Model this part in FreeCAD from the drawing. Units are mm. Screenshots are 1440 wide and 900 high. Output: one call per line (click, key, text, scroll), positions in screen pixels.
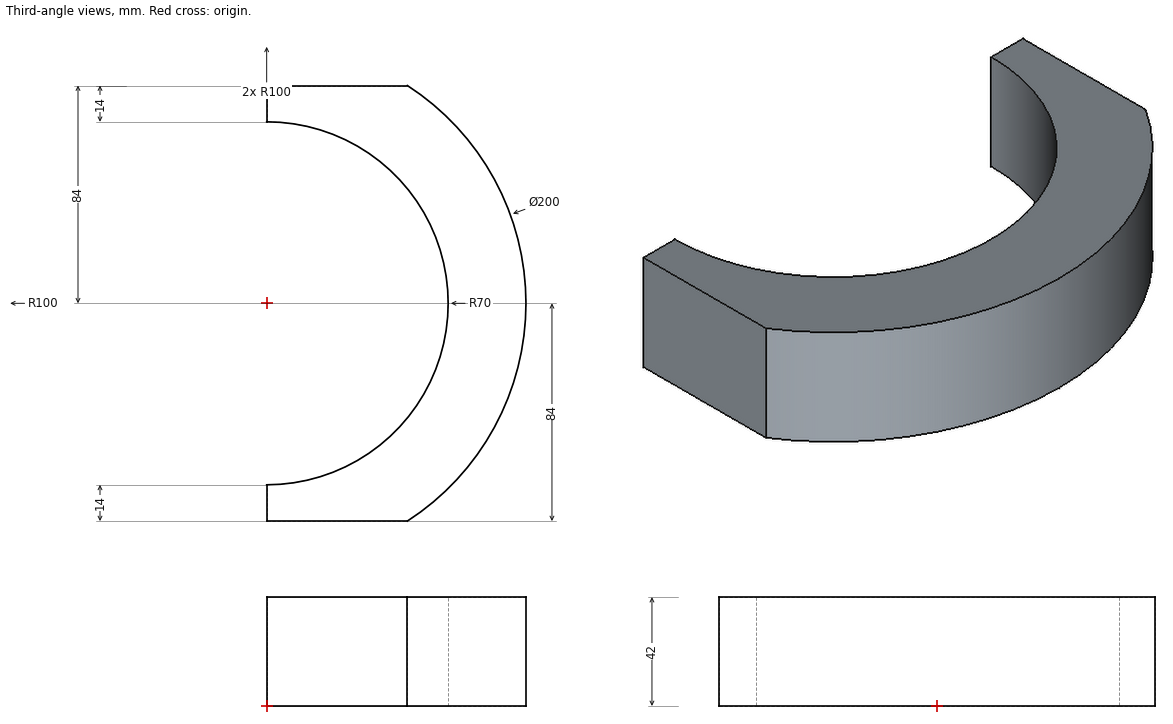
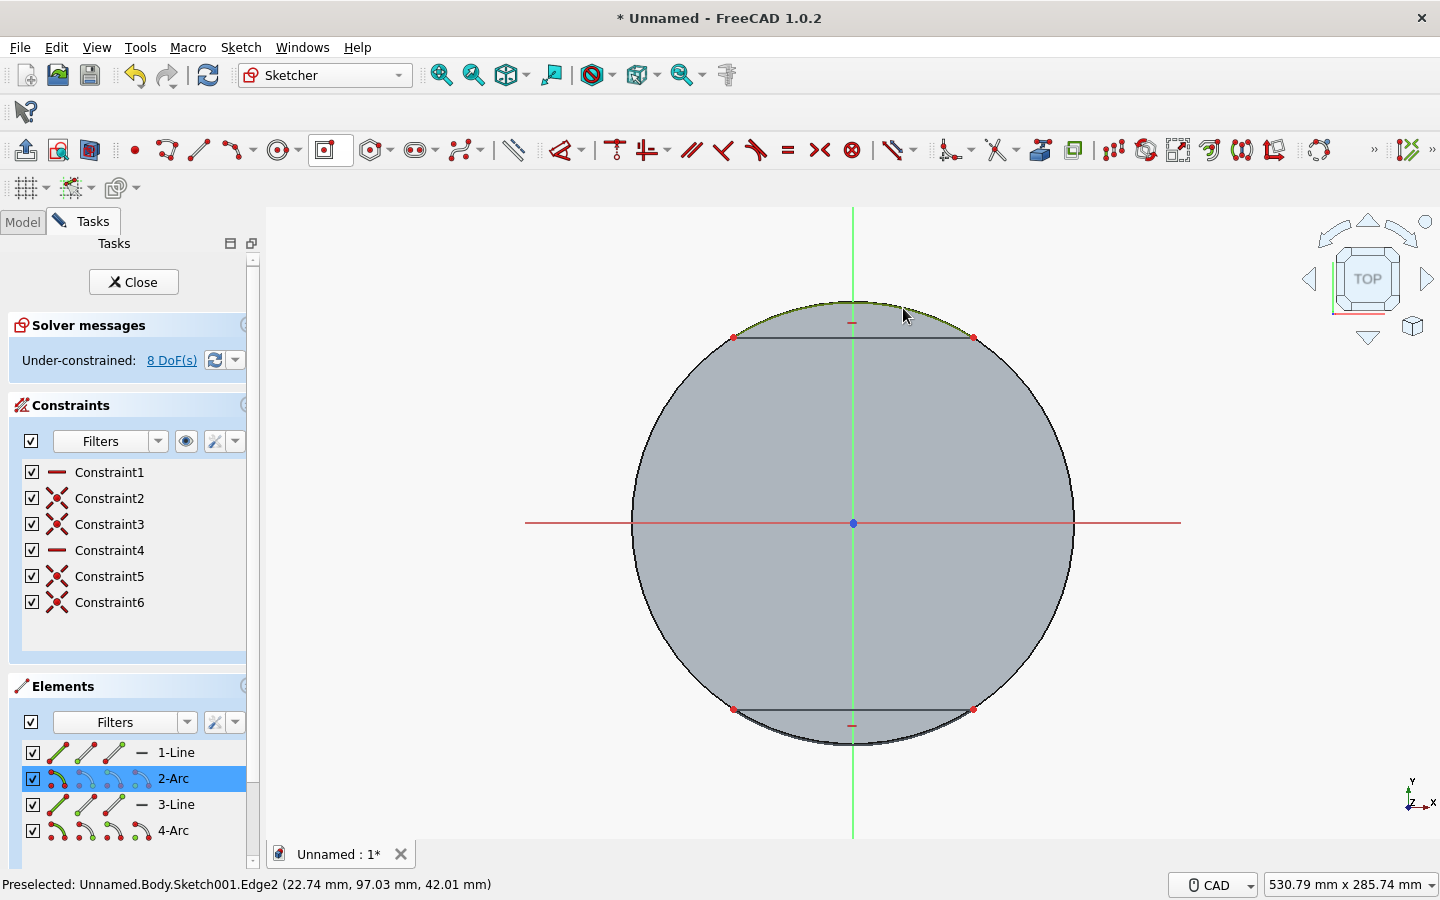
click(803, 740)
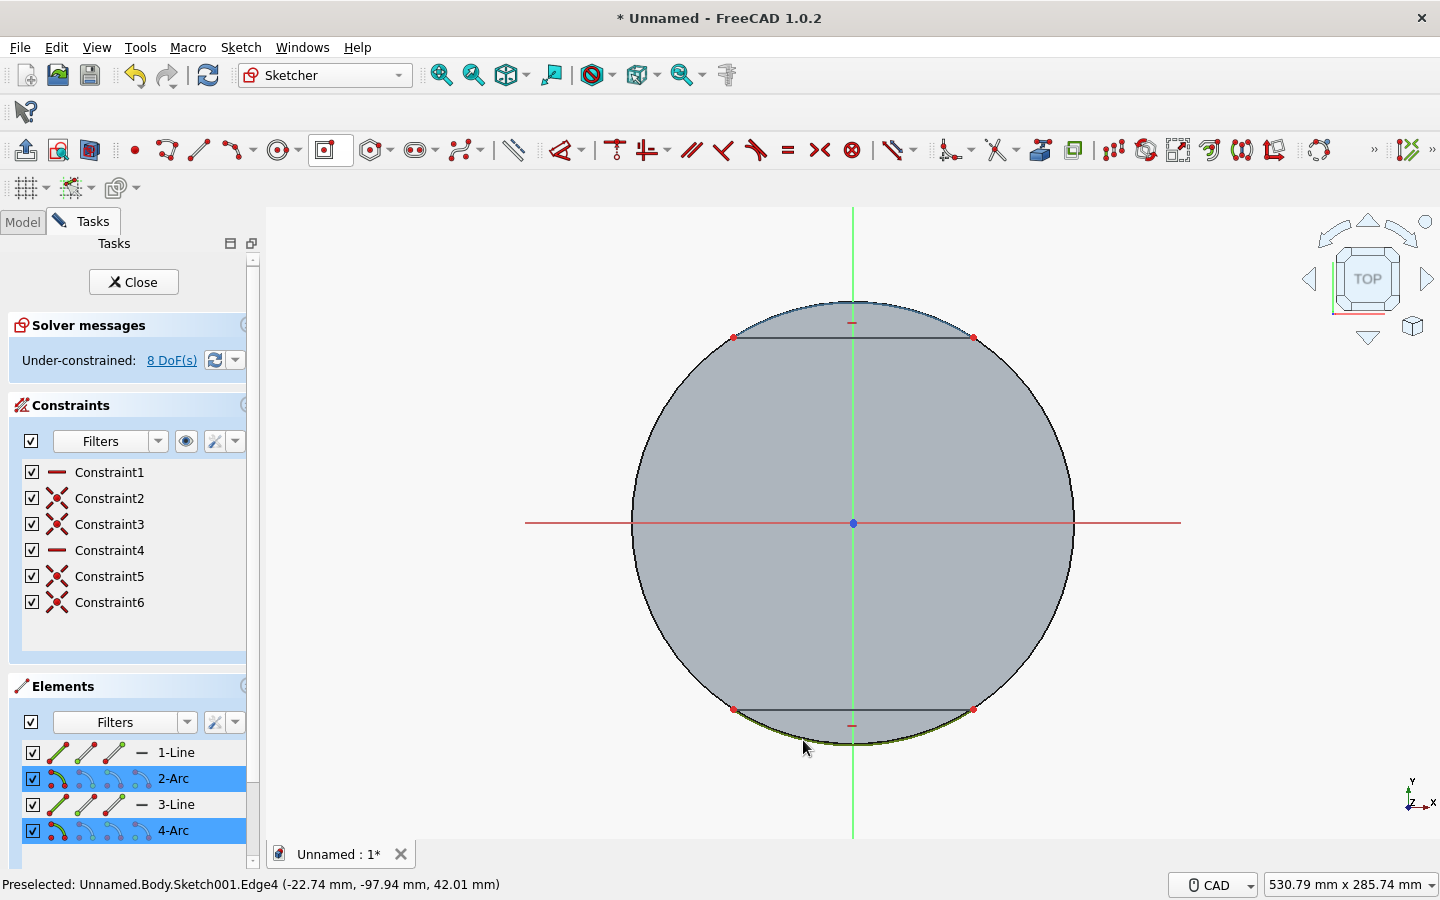
click(616, 150)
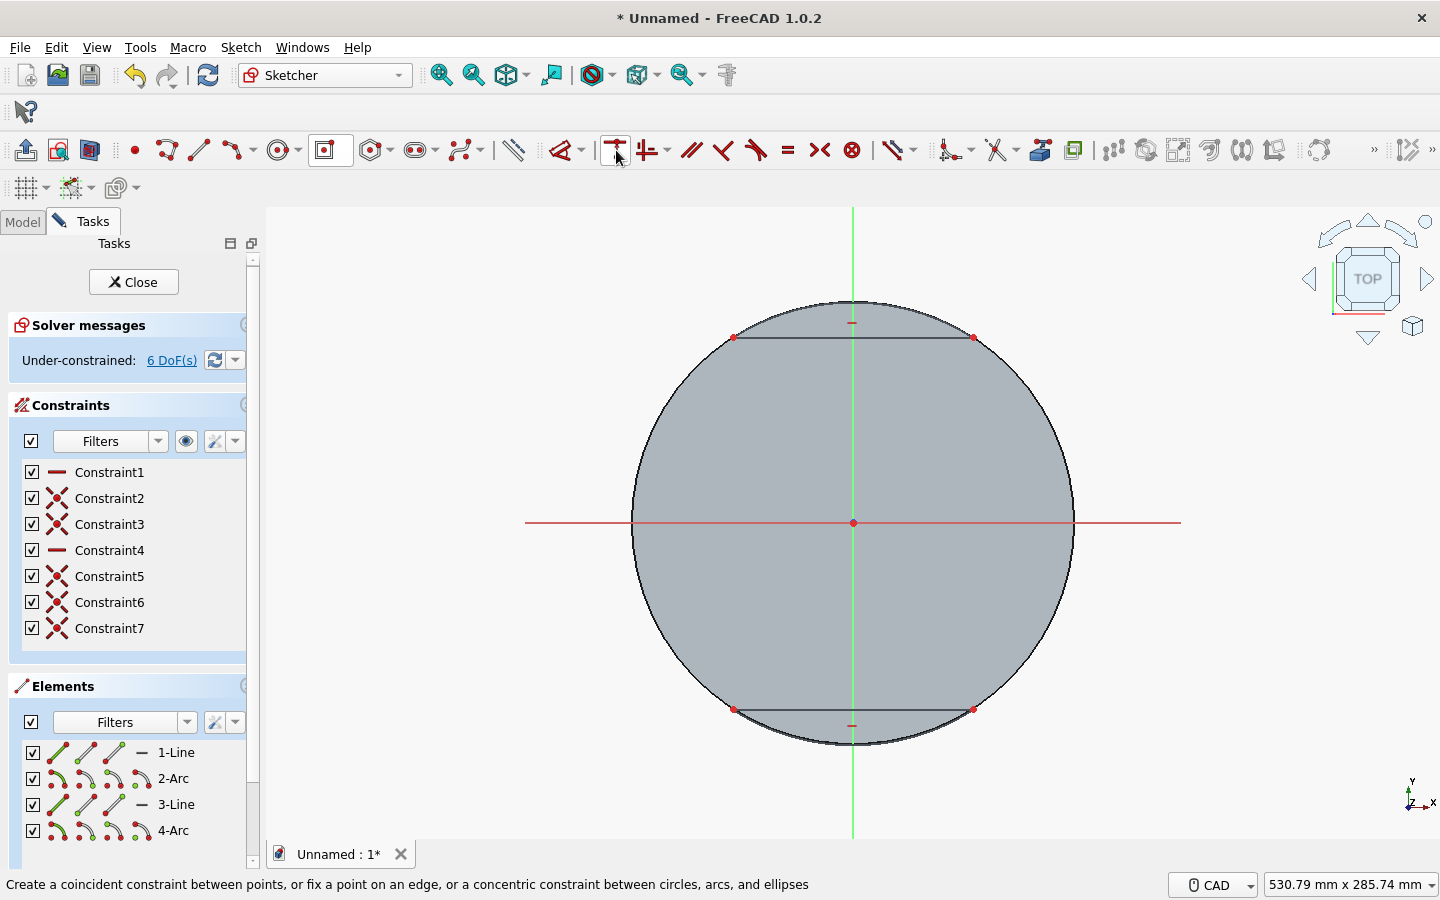
drag(843, 513, 863, 534)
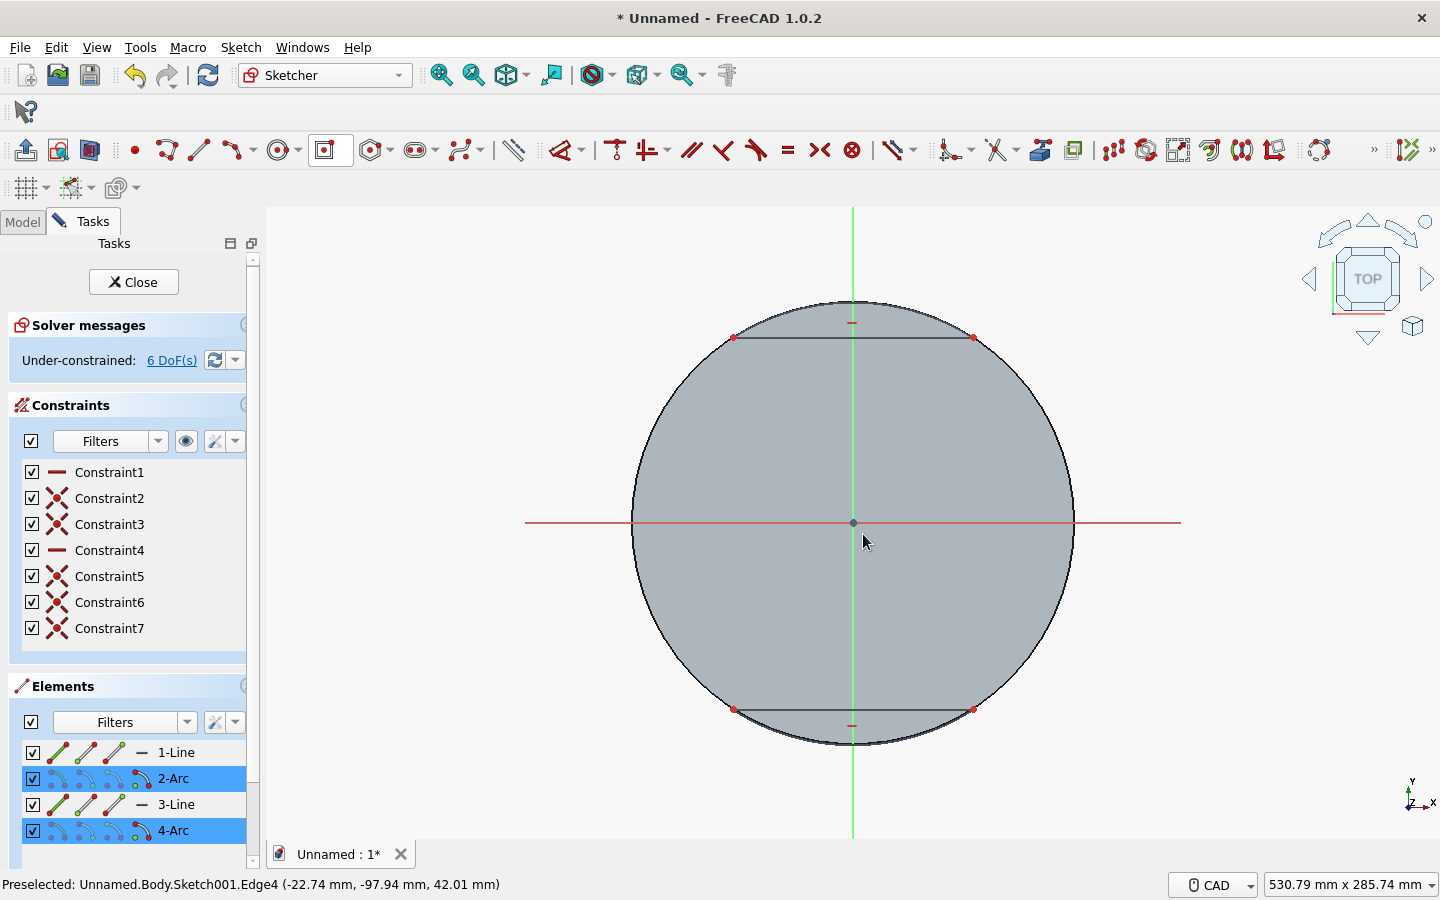
click(616, 150)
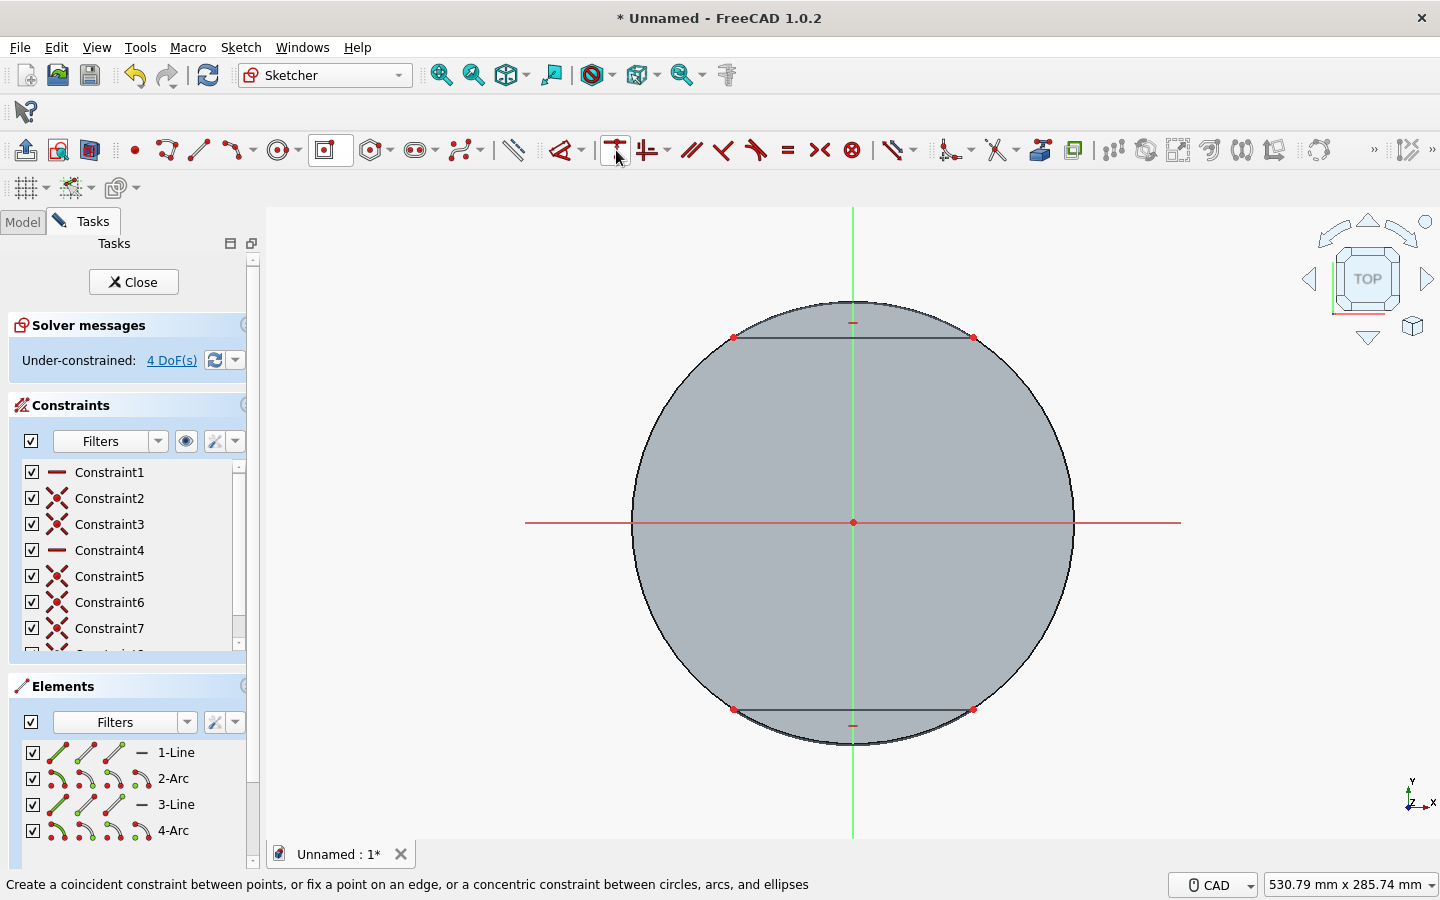
click(903, 308)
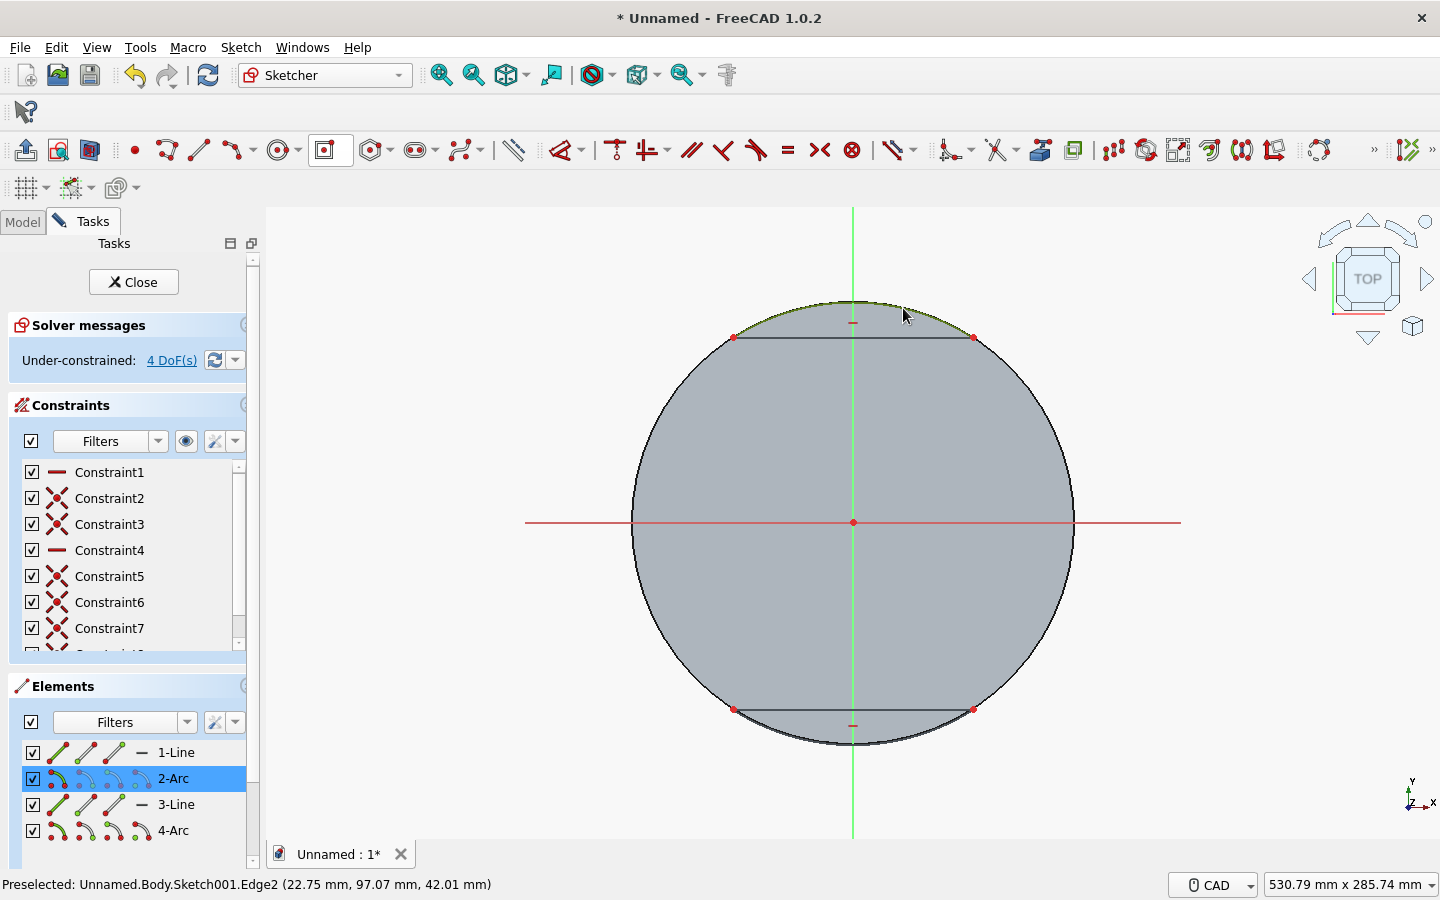
click(803, 739)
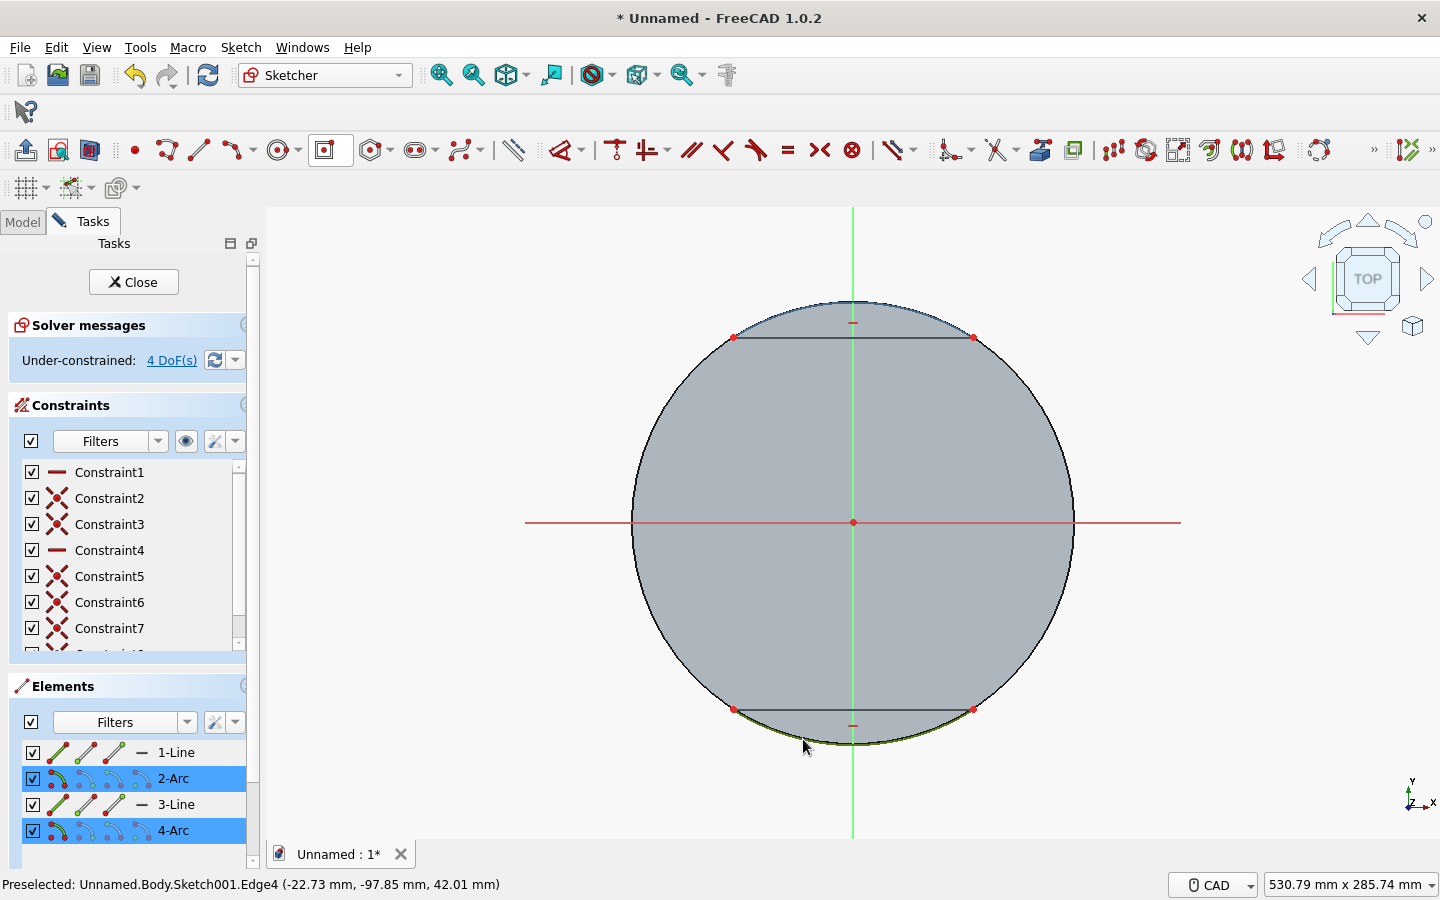
click(788, 150)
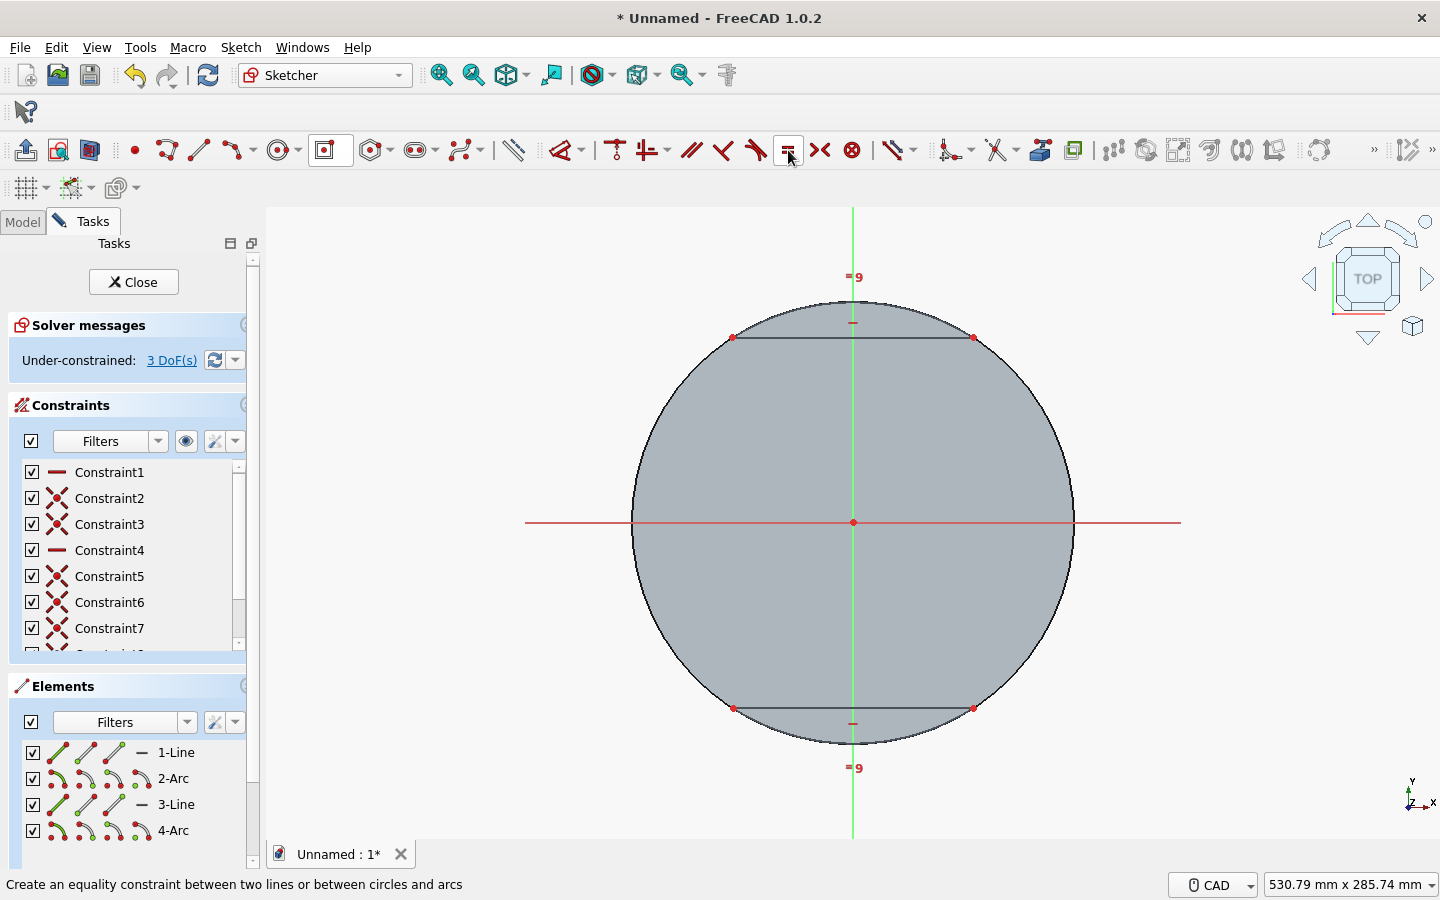
click(560, 150)